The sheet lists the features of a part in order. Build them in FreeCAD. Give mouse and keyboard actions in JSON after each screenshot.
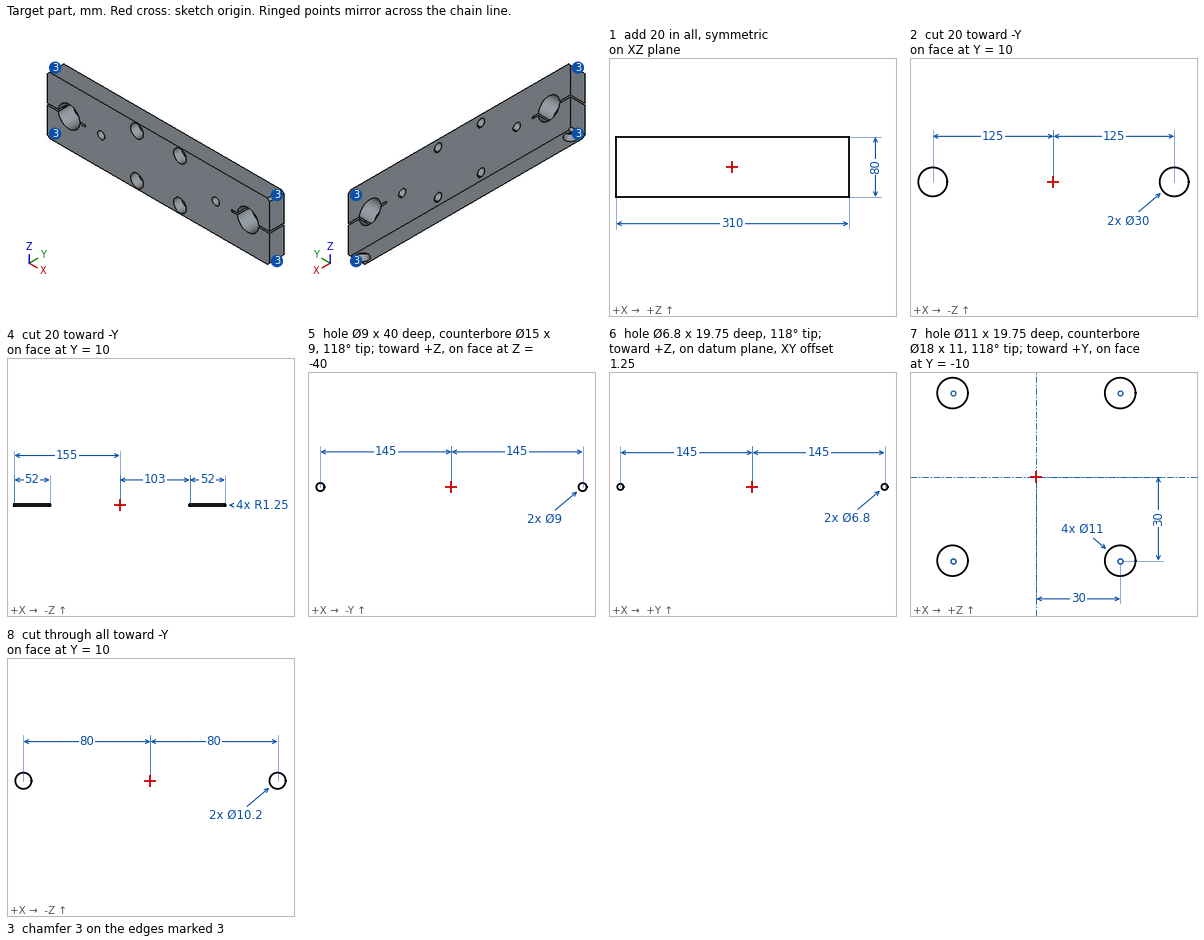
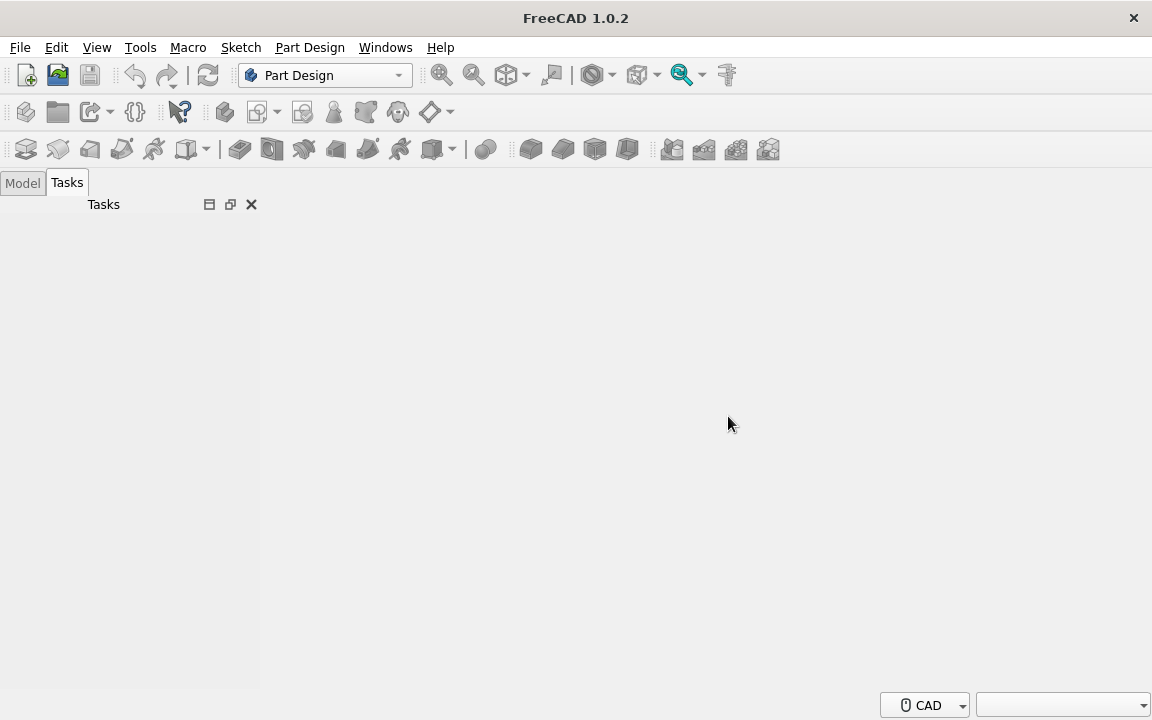
{"action": "left_click", "coordinate": [26, 76]}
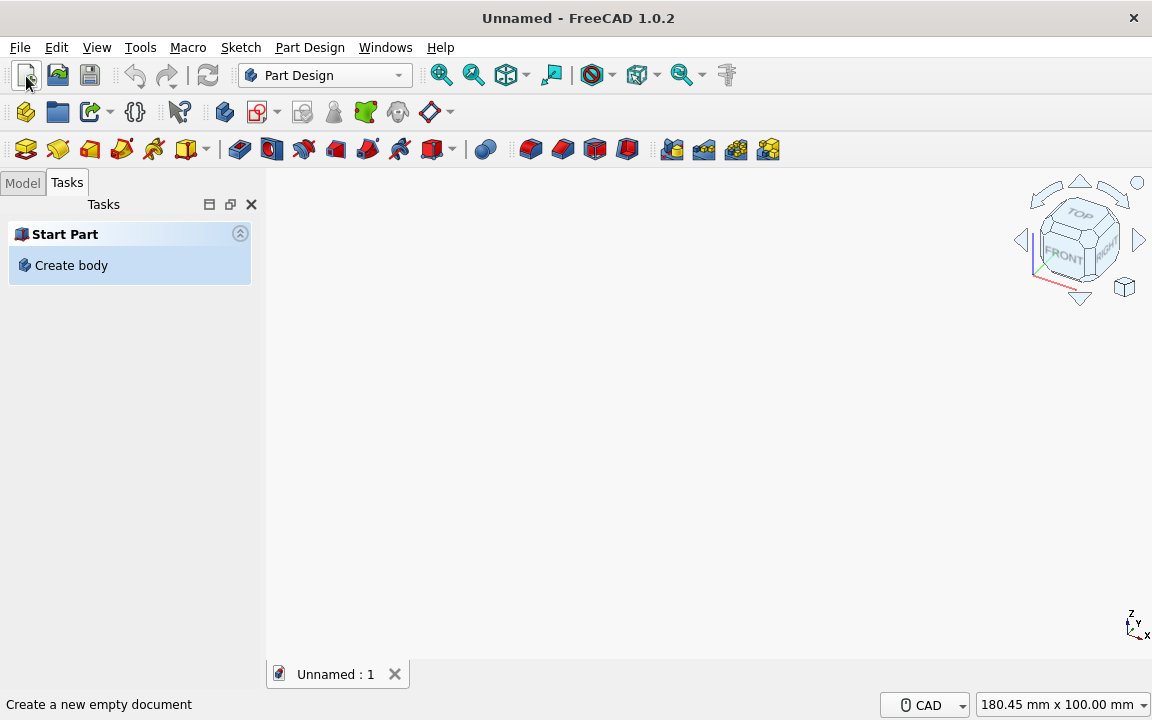
{"action": "left_click", "coordinate": [258, 112]}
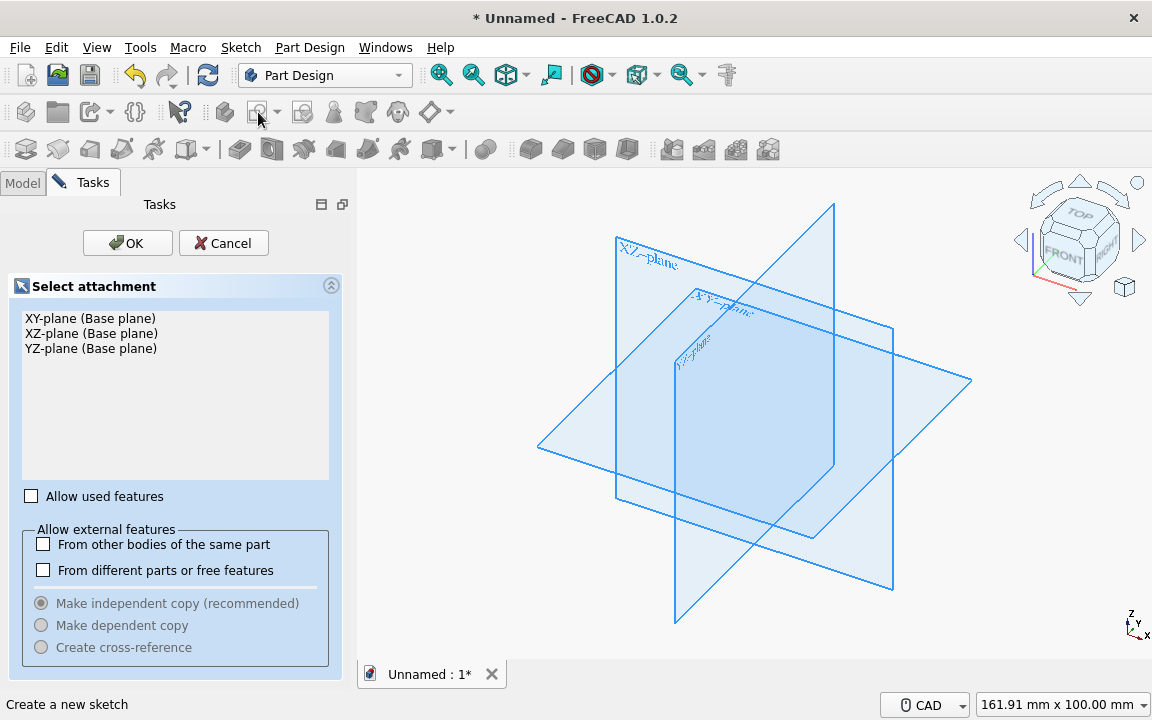
{"action": "left_click", "coordinate": [82, 334]}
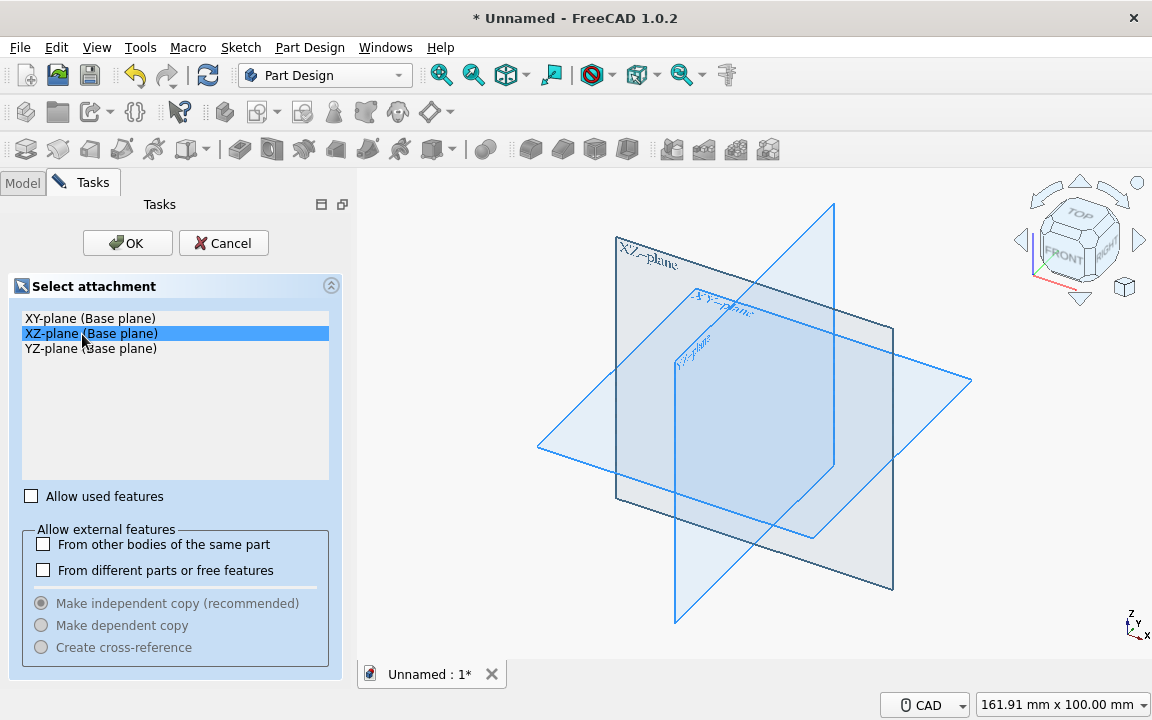
{"action": "left_click", "coordinate": [128, 243]}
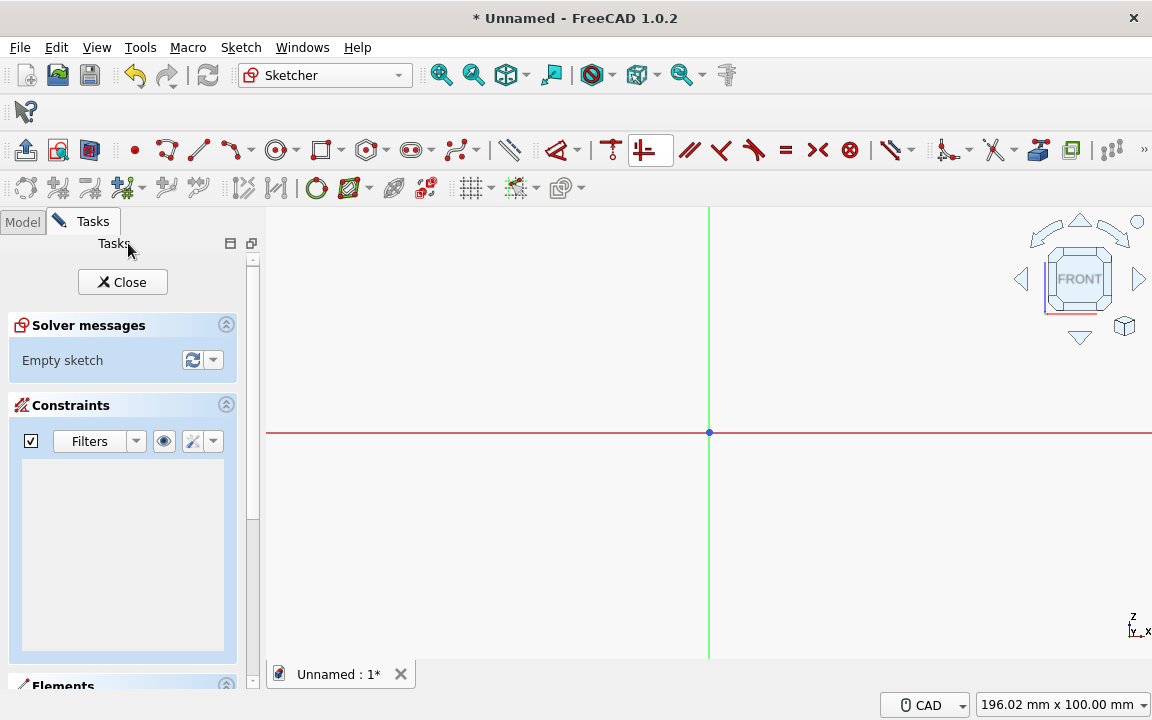
{"action": "scroll", "coordinate": [601, 433], "scroll_direction": "down", "scroll_amount": 5}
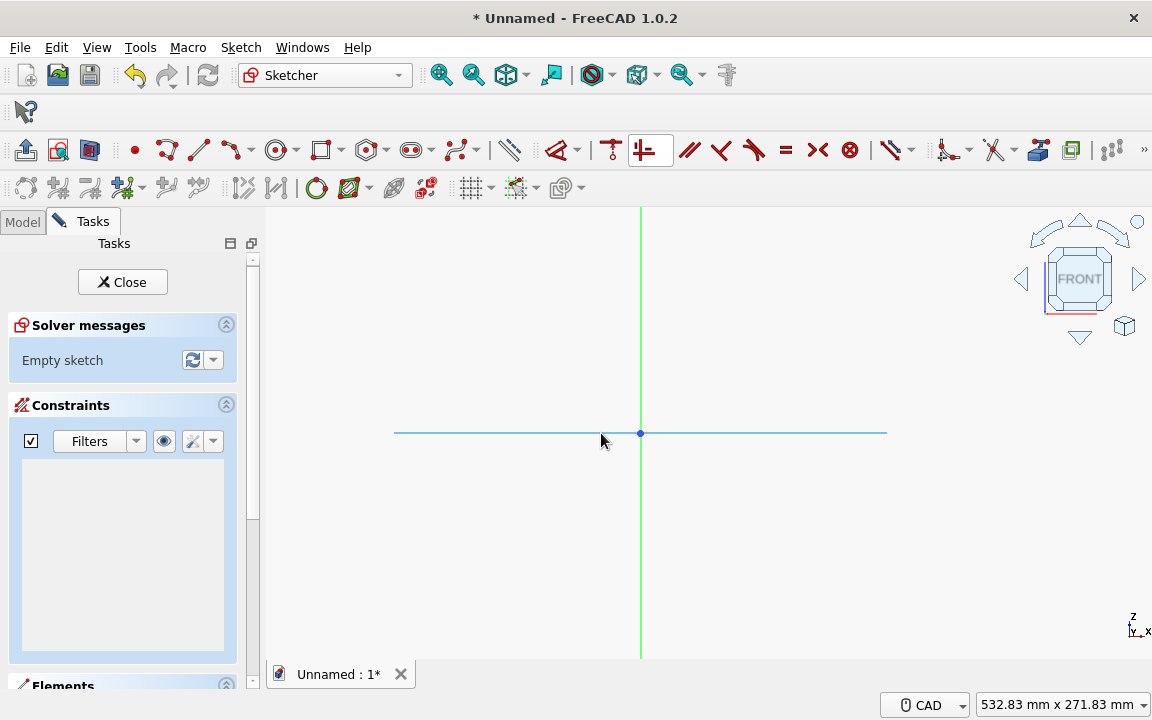
{"action": "left_click", "coordinate": [344, 150]}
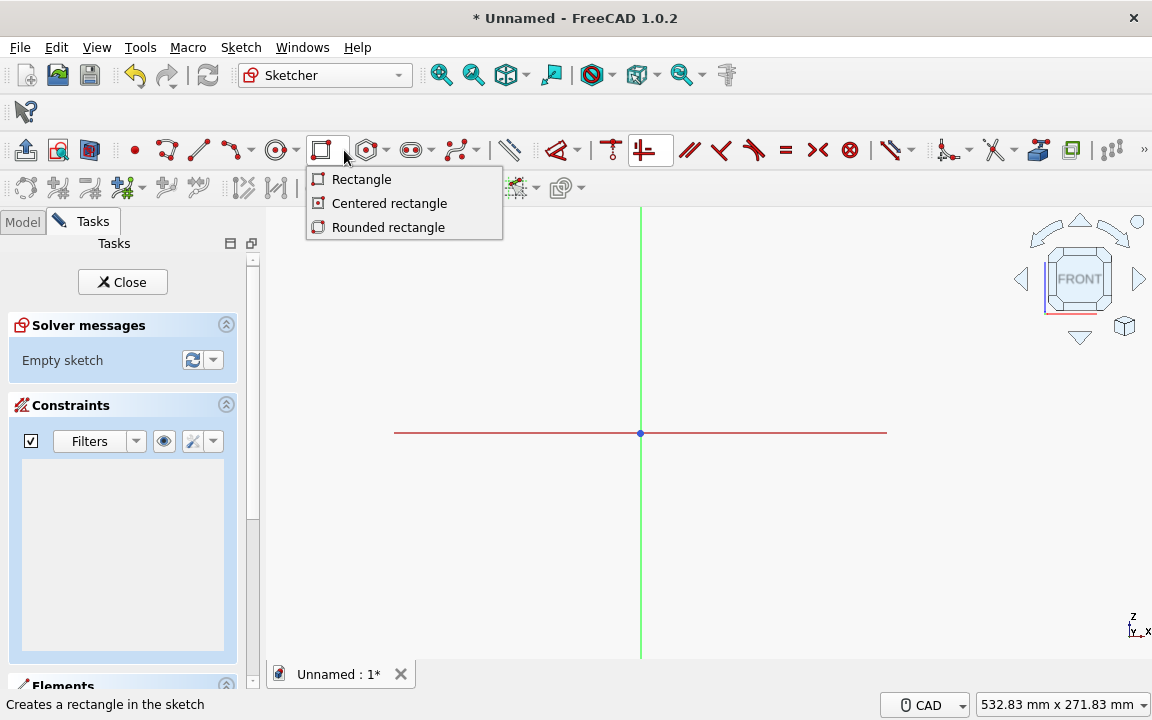
{"action": "left_click", "coordinate": [404, 203]}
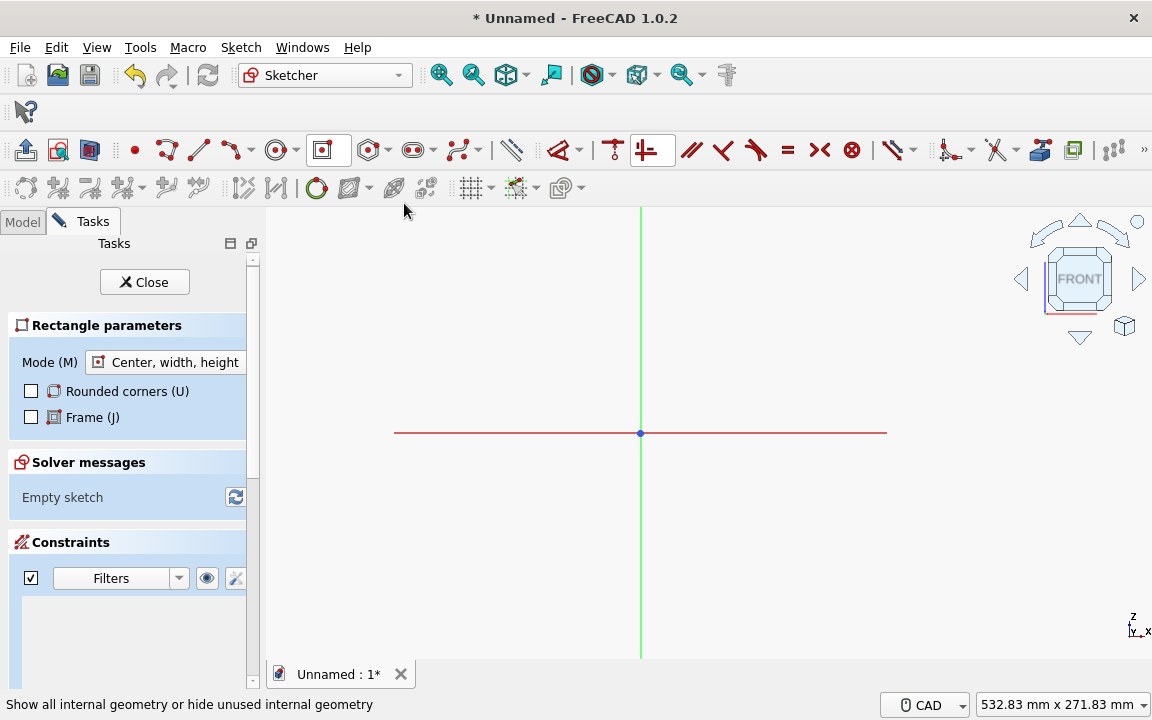
{"action": "left_click", "coordinate": [641, 433]}
{"action": "mouse_move", "coordinate": [899, 367]}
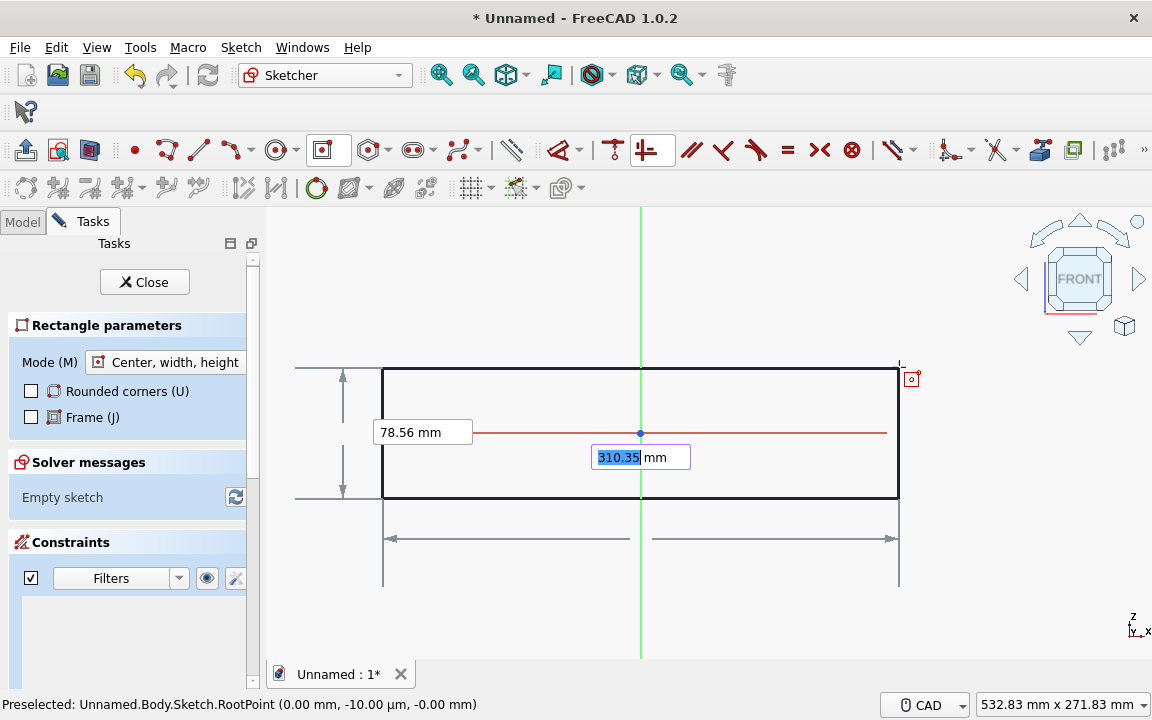
{"action": "type", "text": "310"}
{"action": "key", "text": "Tab"}
{"action": "type", "text": "80"}
{"action": "key", "text": "Return"}
{"action": "key", "text": "Escape"}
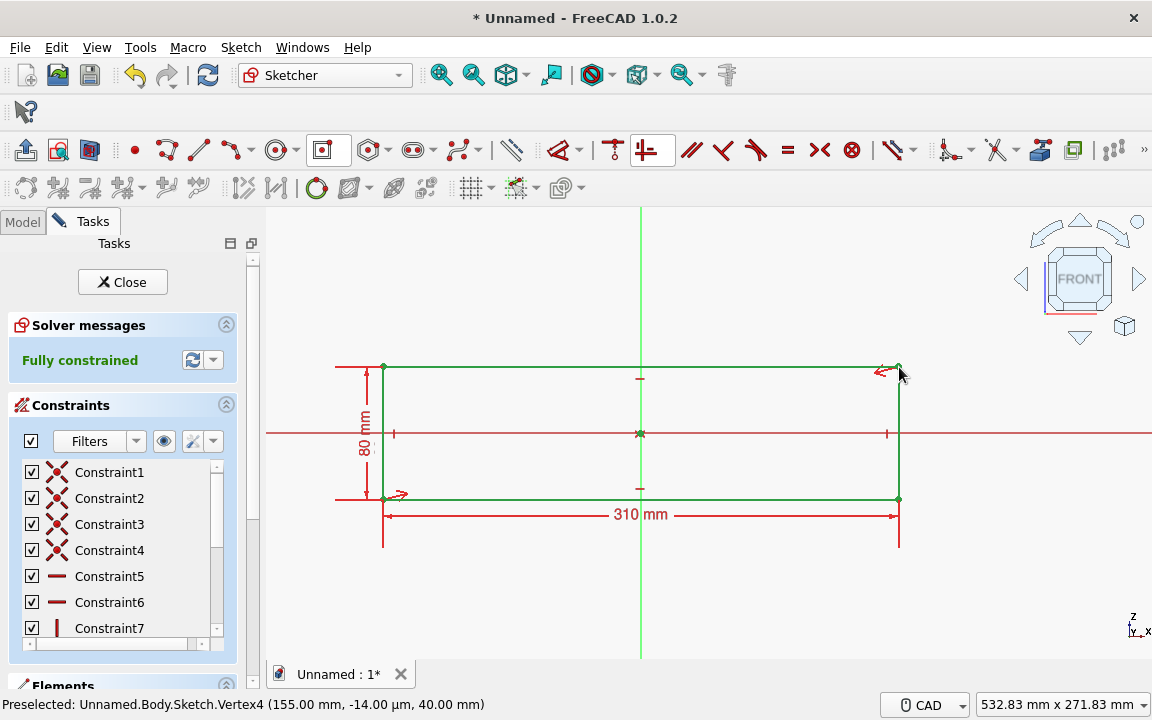
{"action": "left_click", "coordinate": [123, 282]}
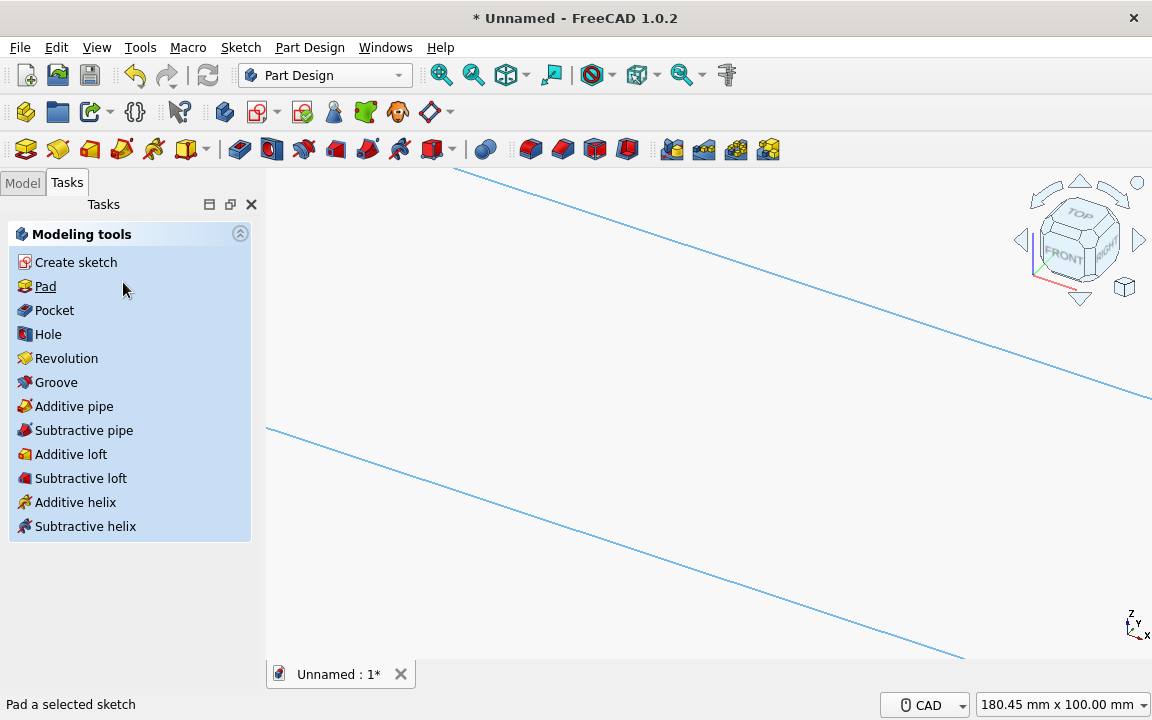
{"action": "left_click", "coordinate": [26, 150]}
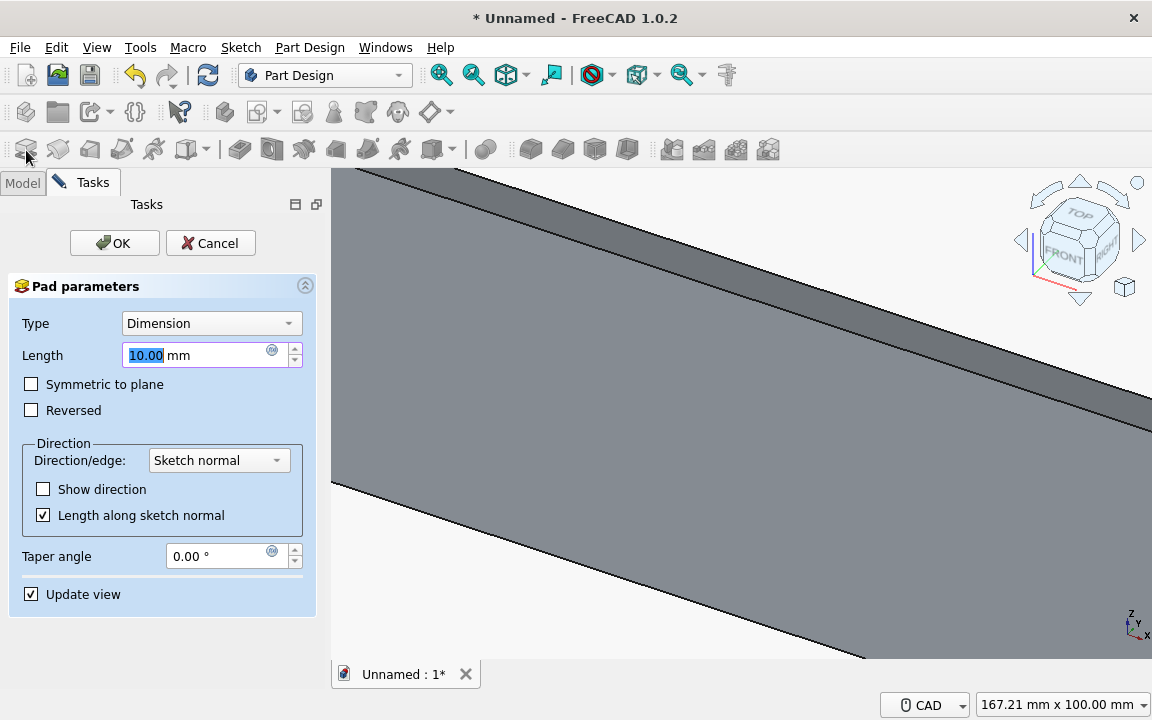
{"action": "type", "text": "20"}
{"action": "key", "text": "Tab"}